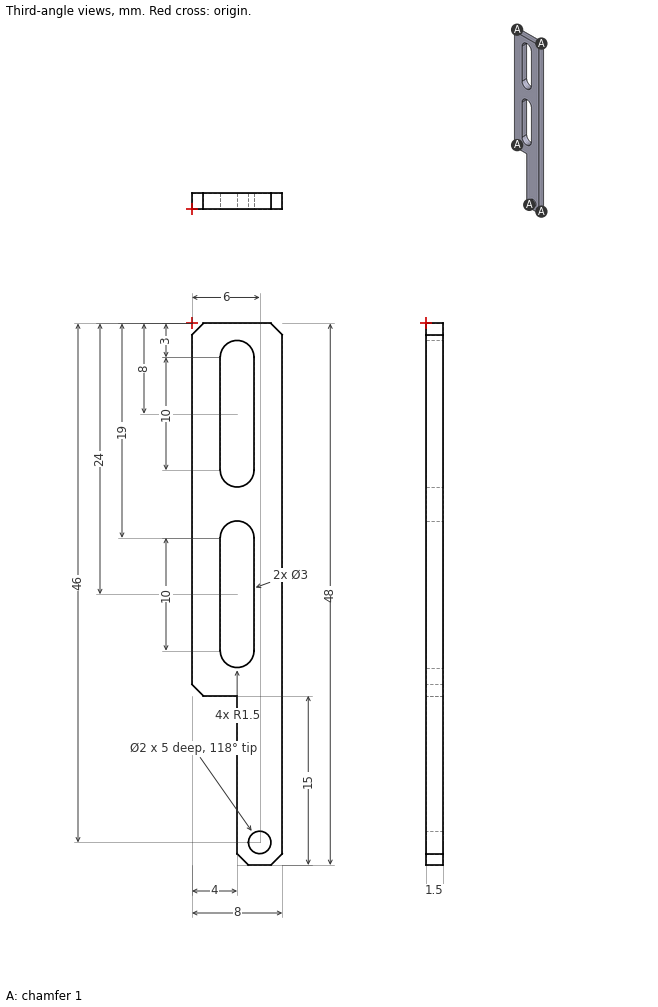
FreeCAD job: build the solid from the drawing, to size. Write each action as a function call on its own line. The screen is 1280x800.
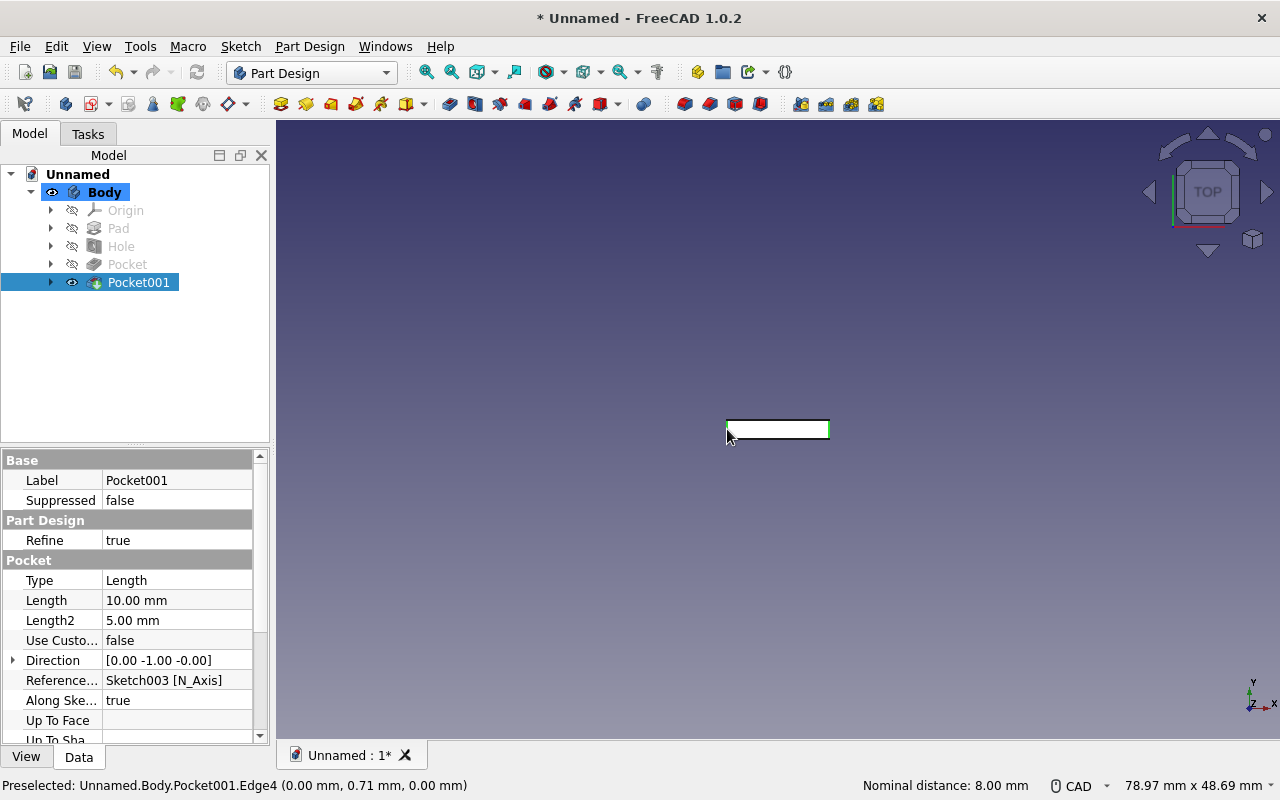
key(1)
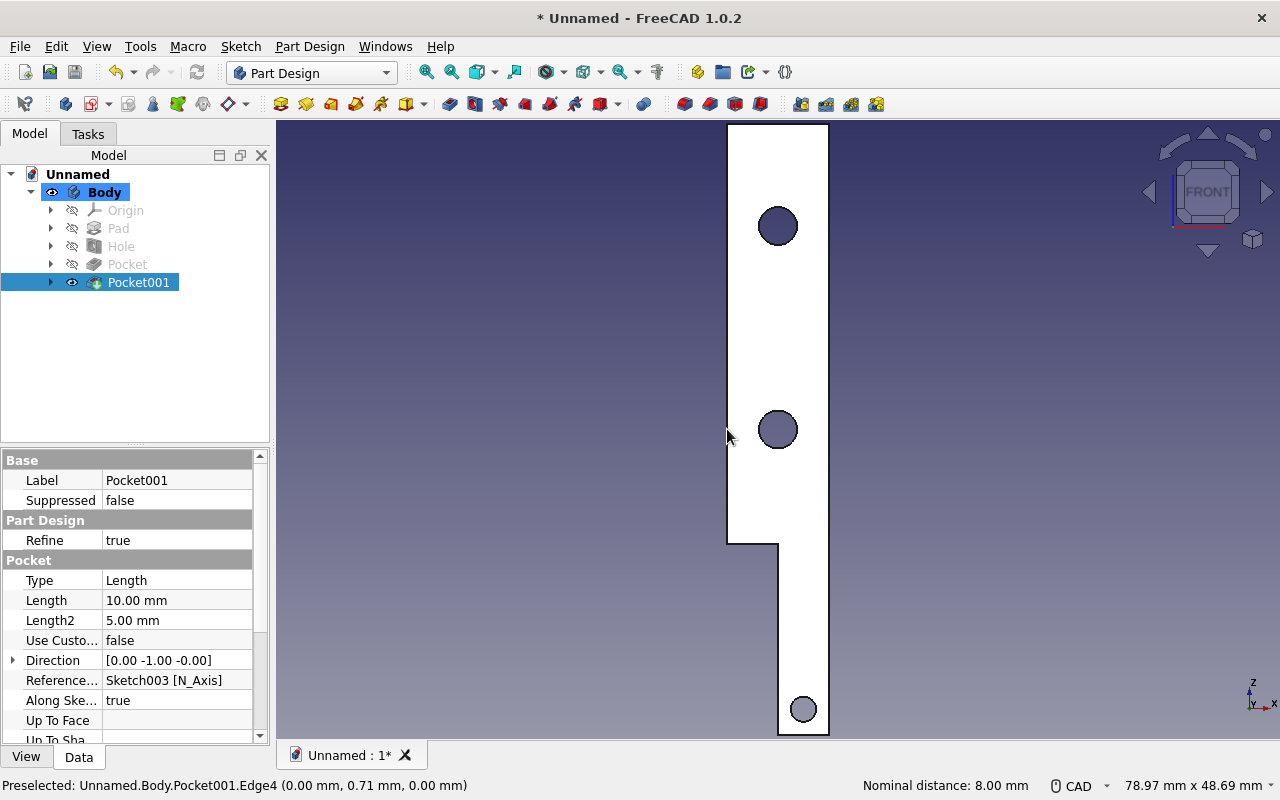
scroll(727, 543, up, 4)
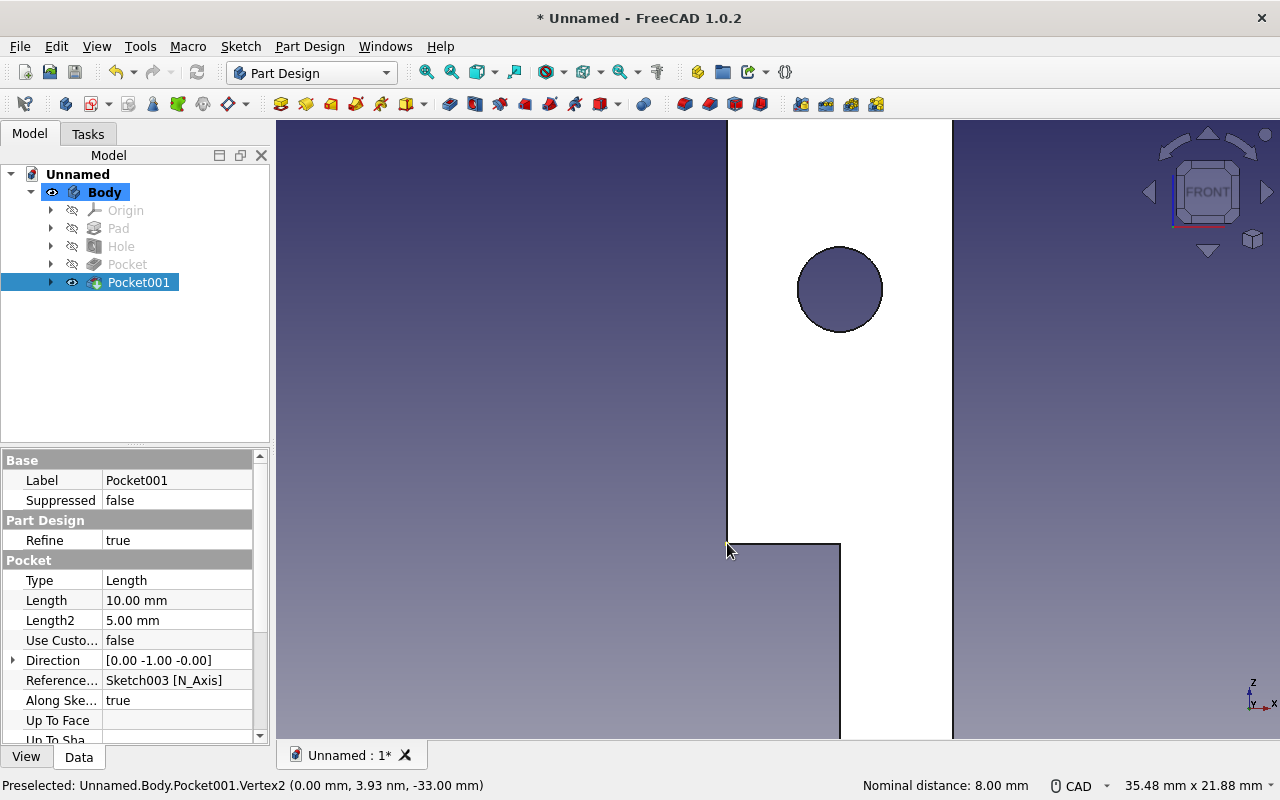
key(v)
key(f)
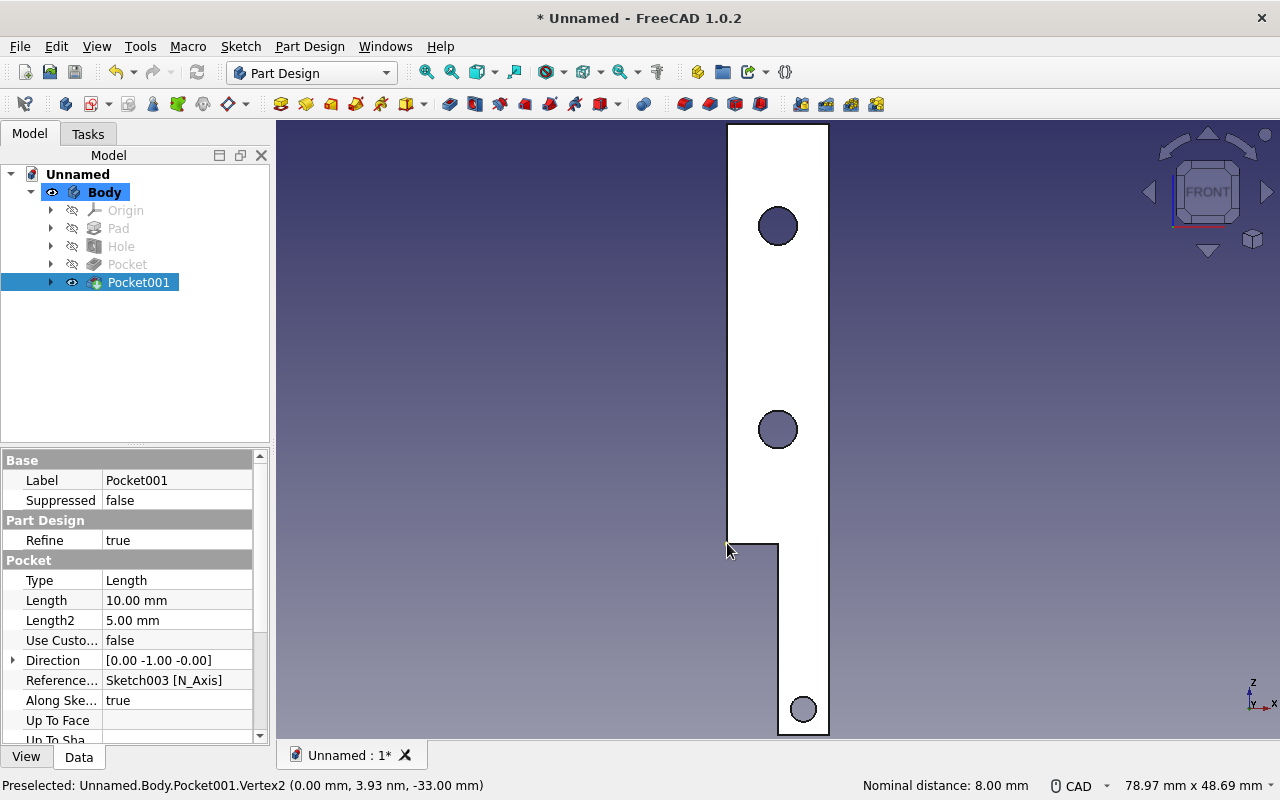
key(3)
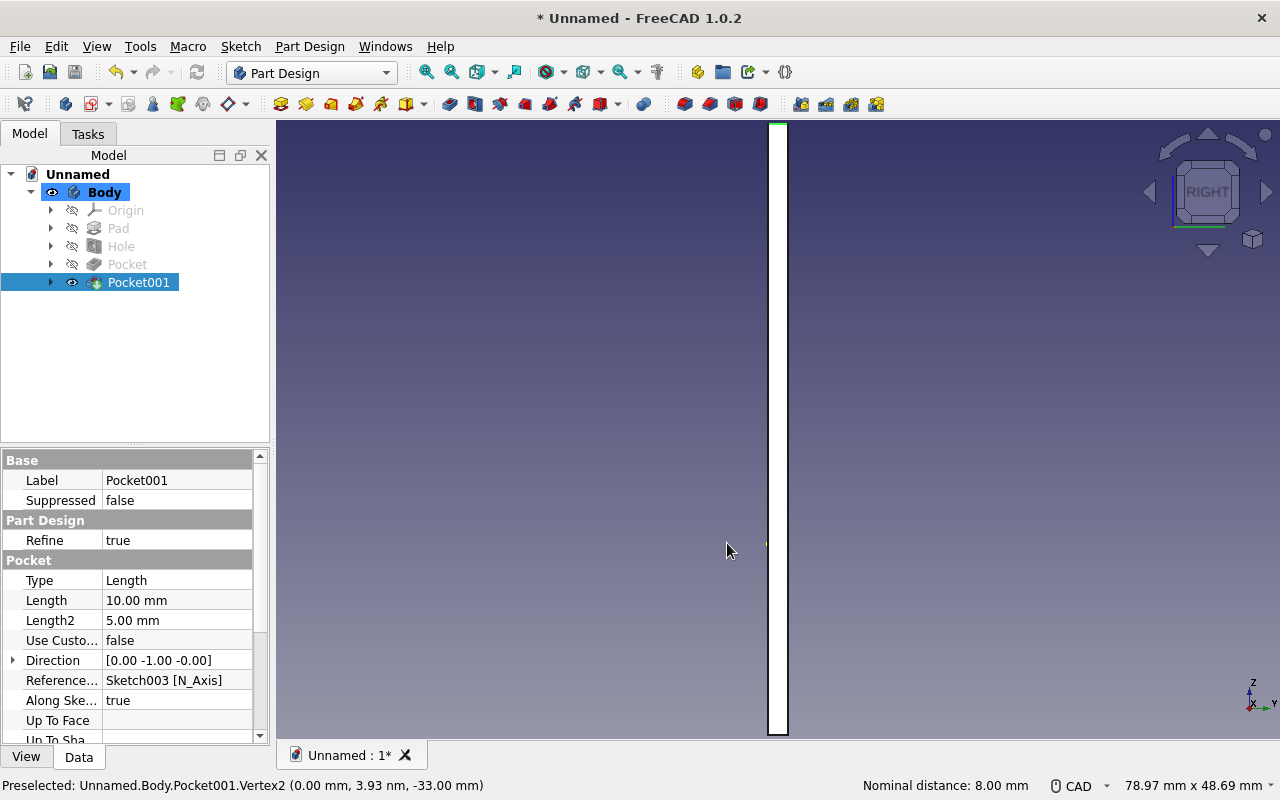
scroll(778, 543, up, 4)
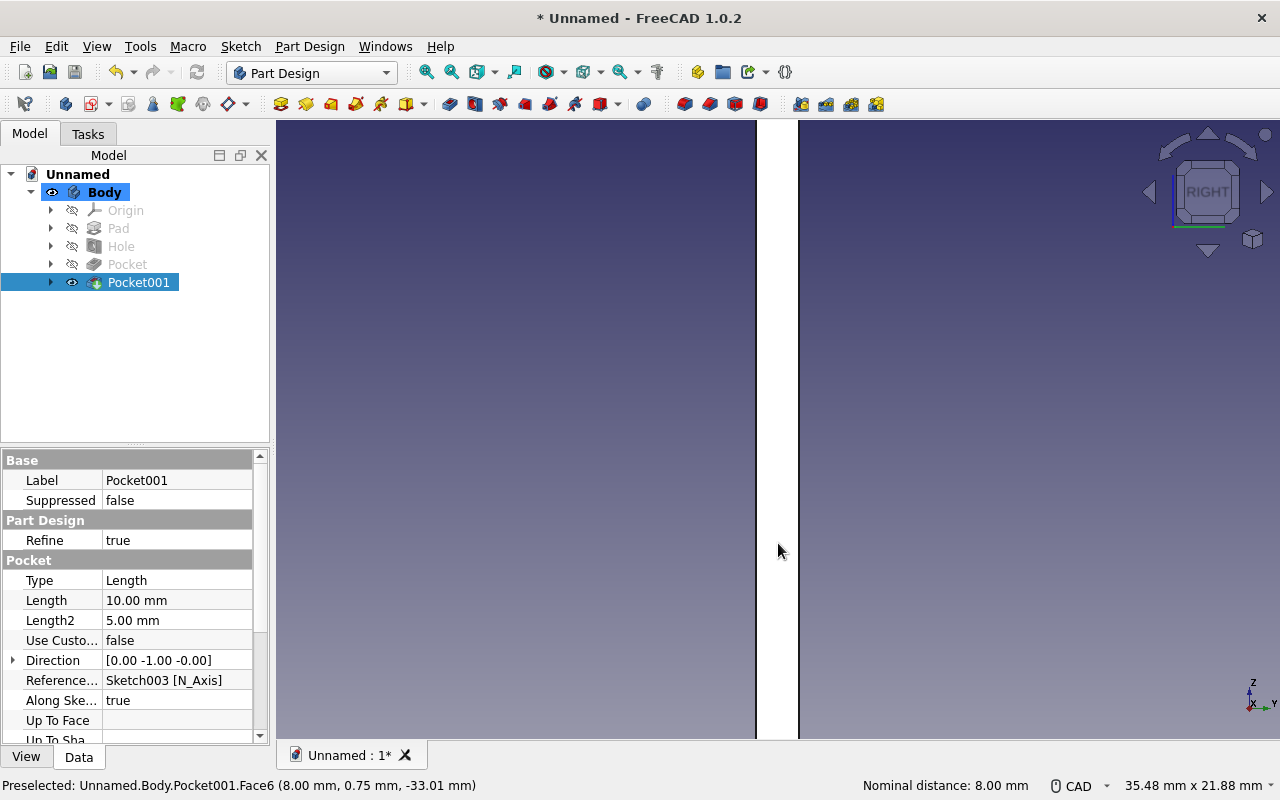
click(427, 72)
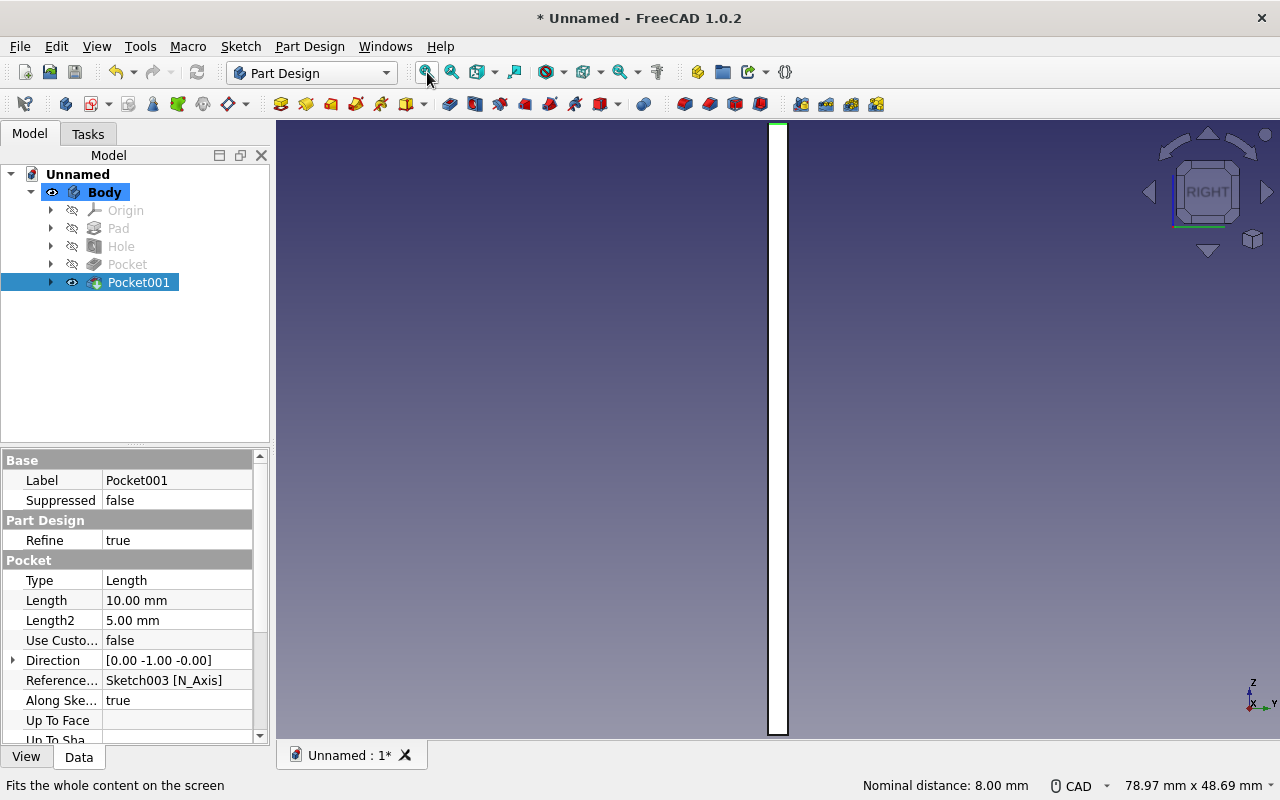
key(5)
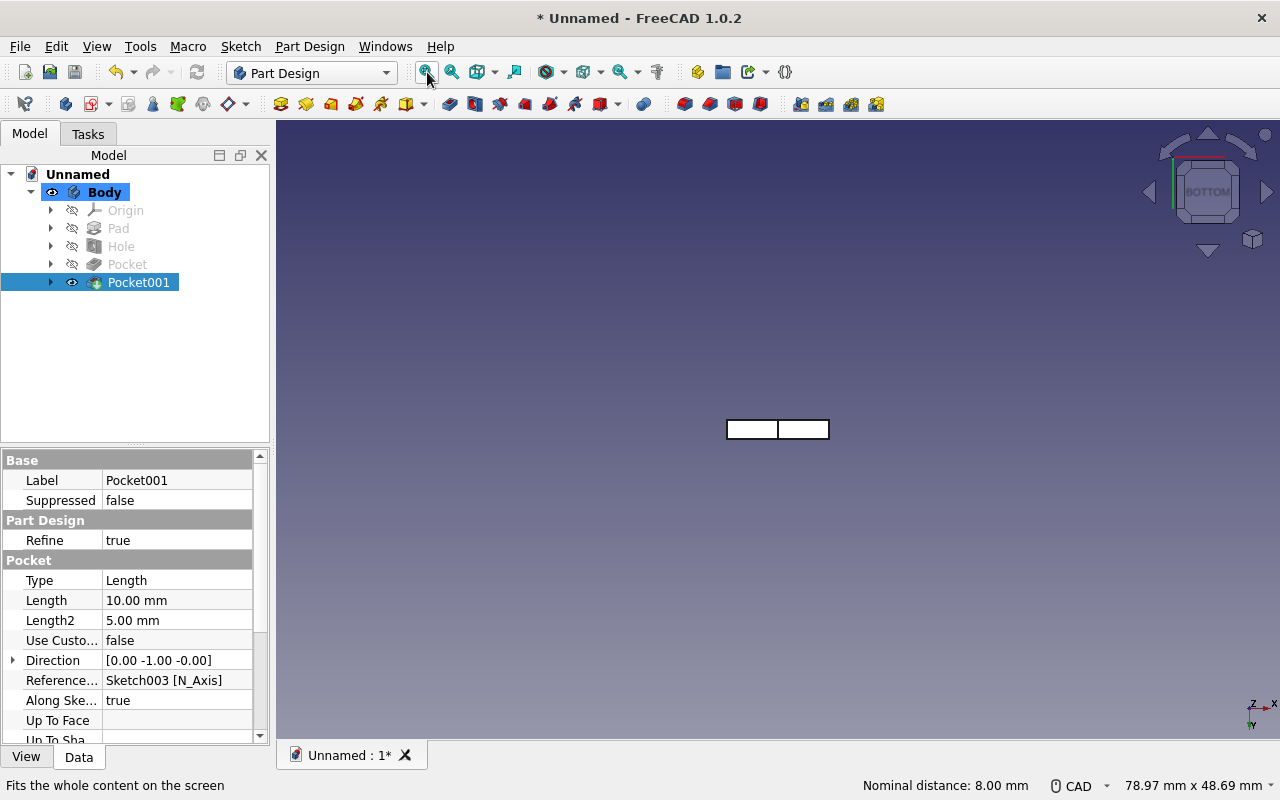
key(v)
key(f)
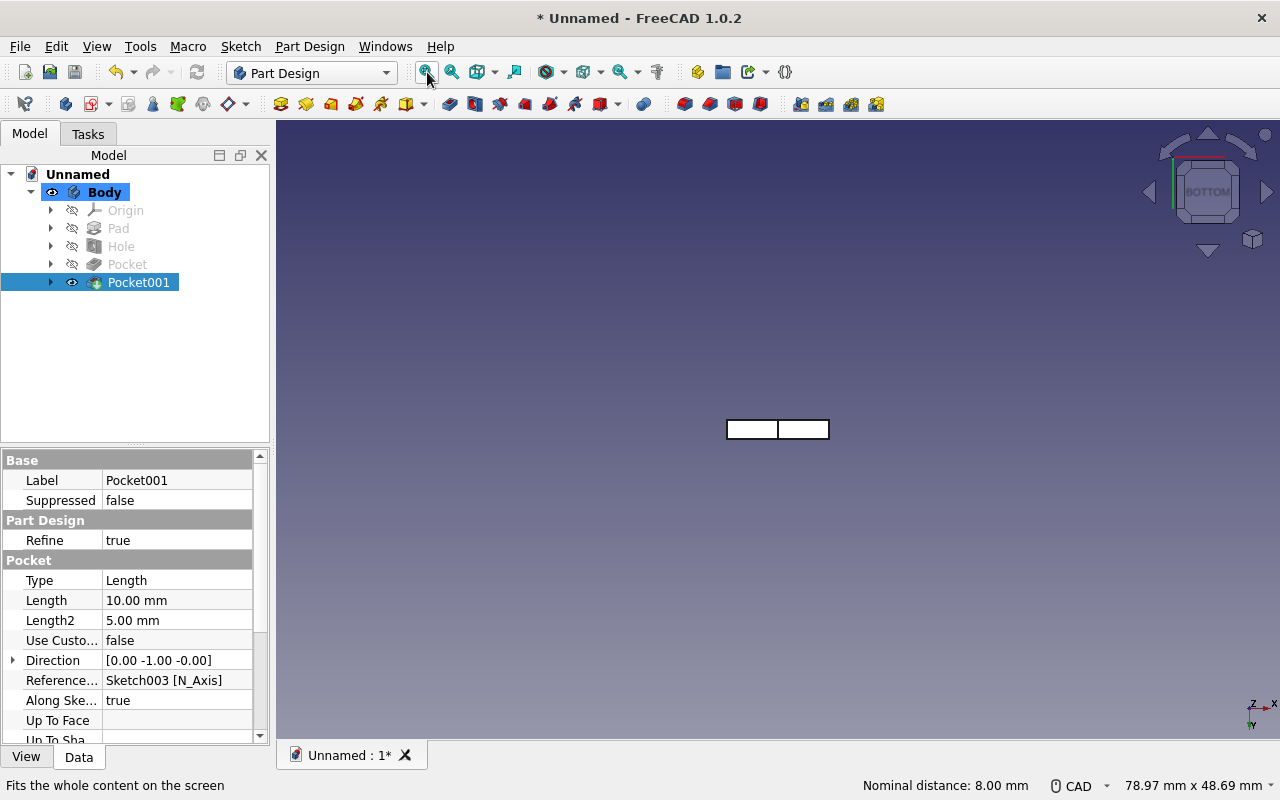
click(727, 428, ctrl)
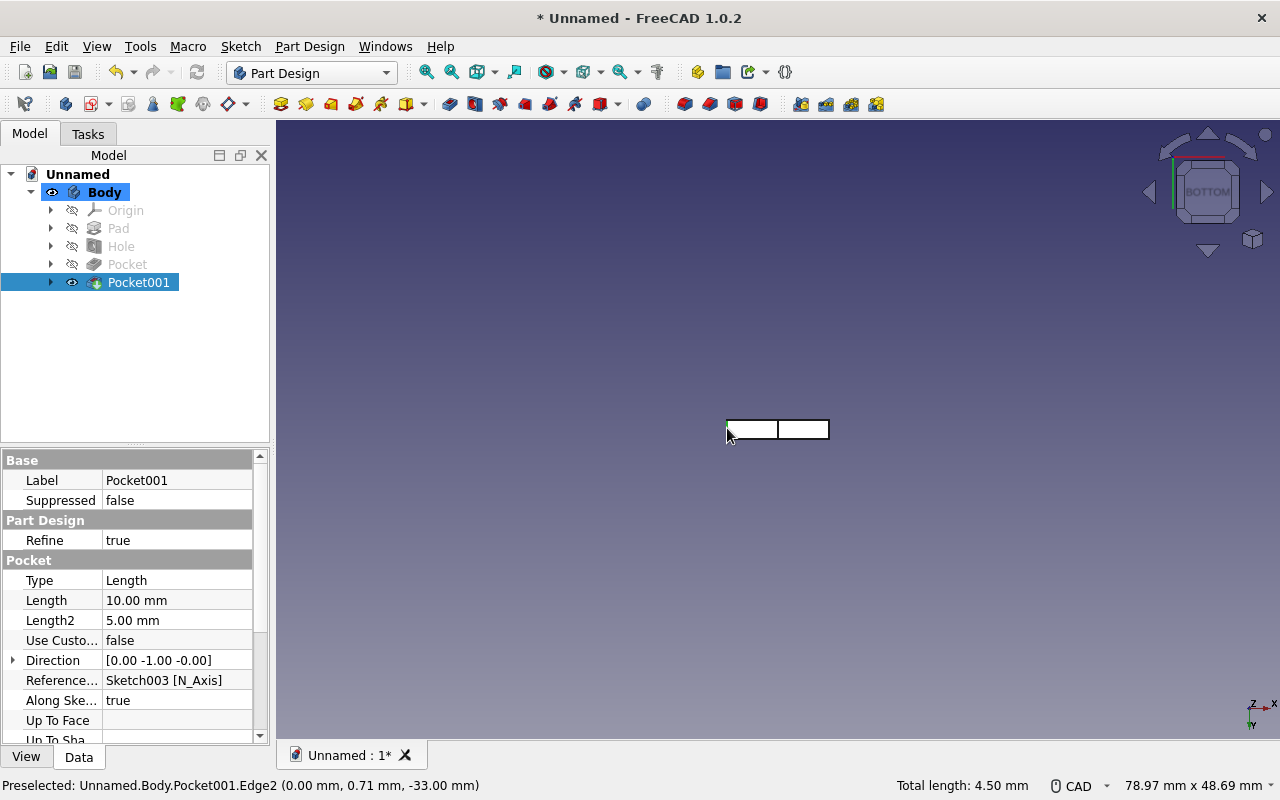
click(778, 428, ctrl)